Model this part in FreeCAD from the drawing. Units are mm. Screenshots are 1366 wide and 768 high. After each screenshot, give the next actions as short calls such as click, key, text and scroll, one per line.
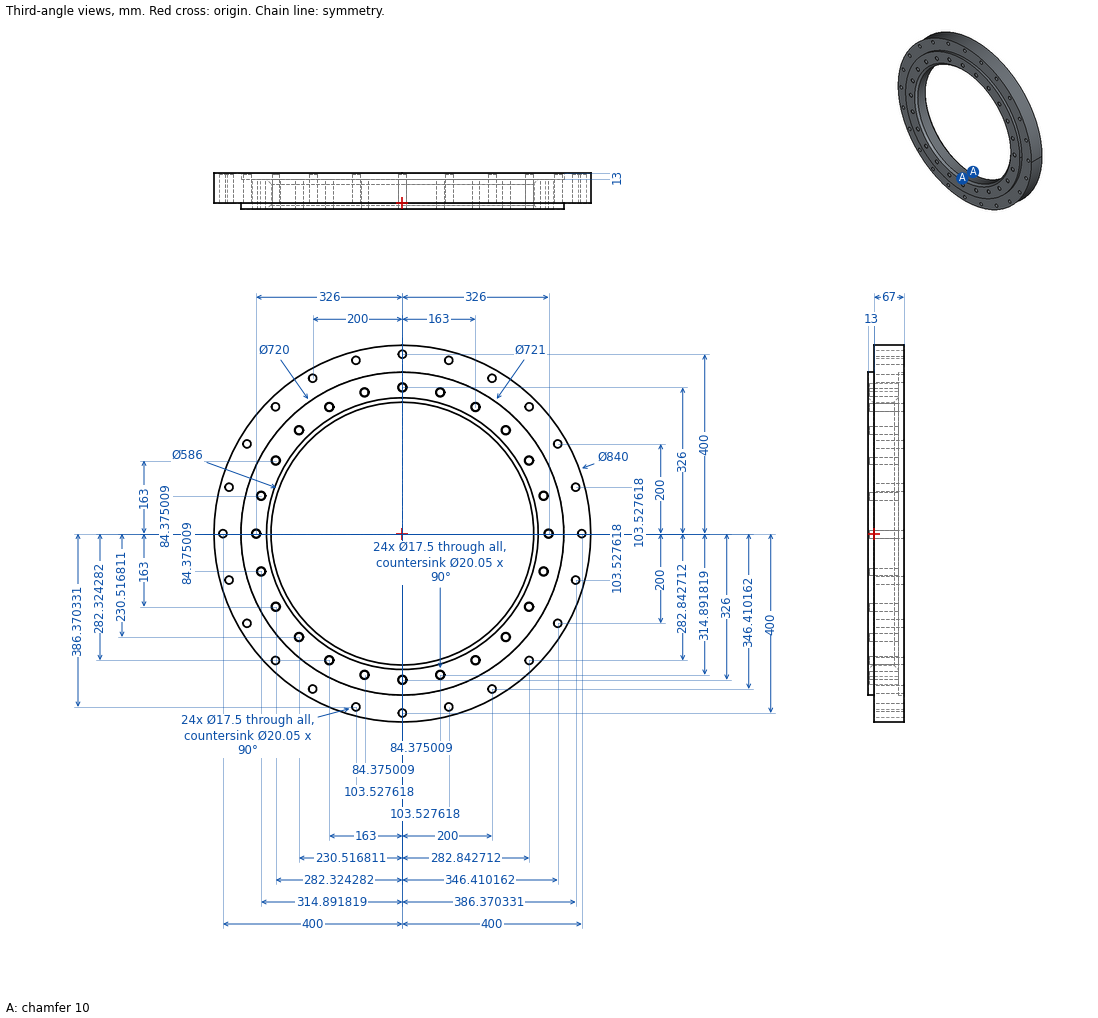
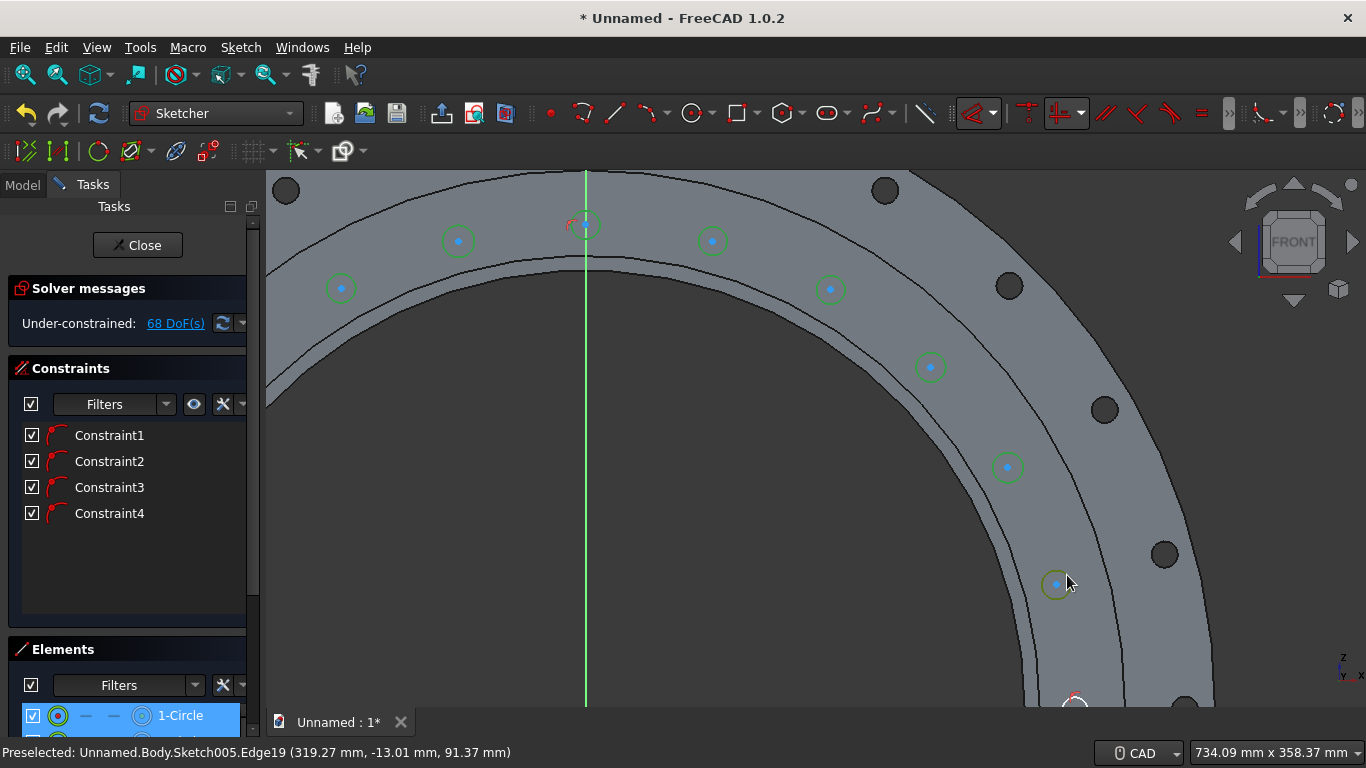
scroll(842, 281, down, 5)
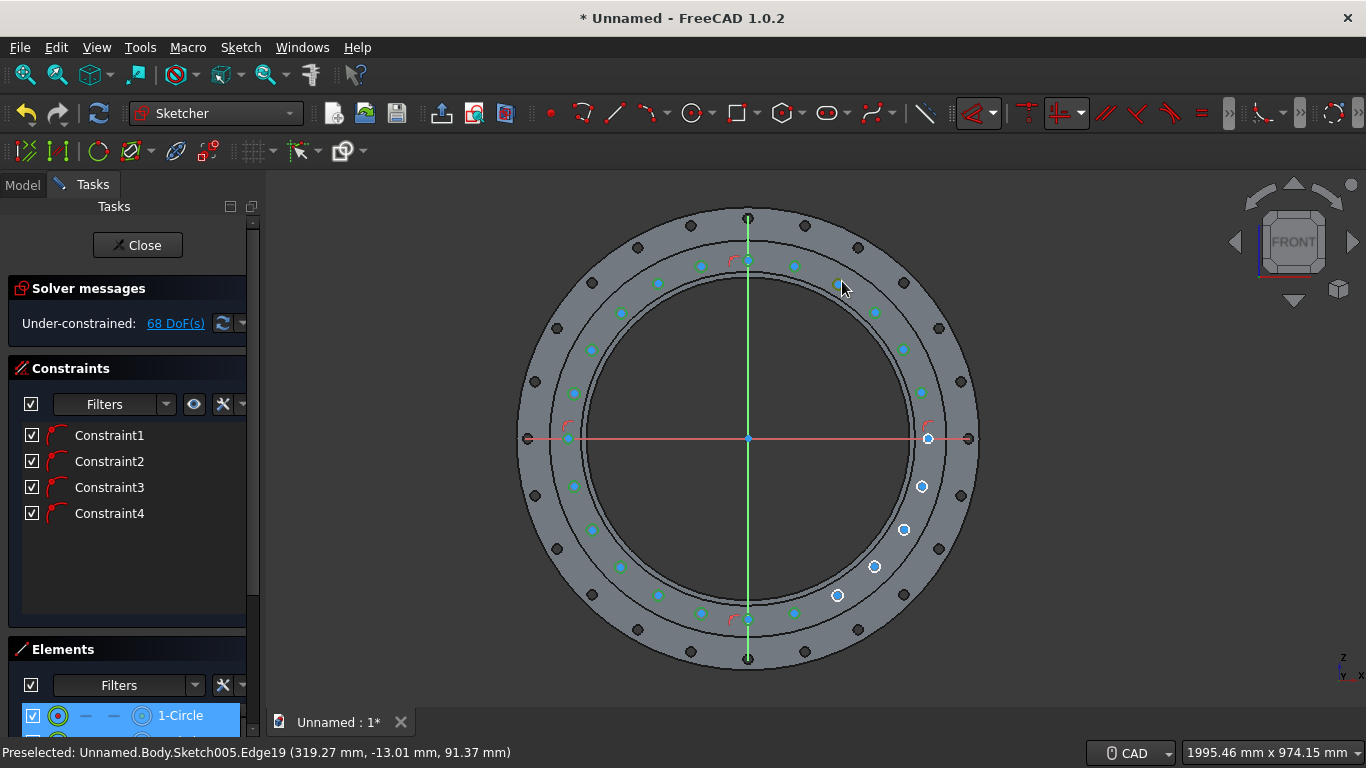
scroll(928, 434, up, 6)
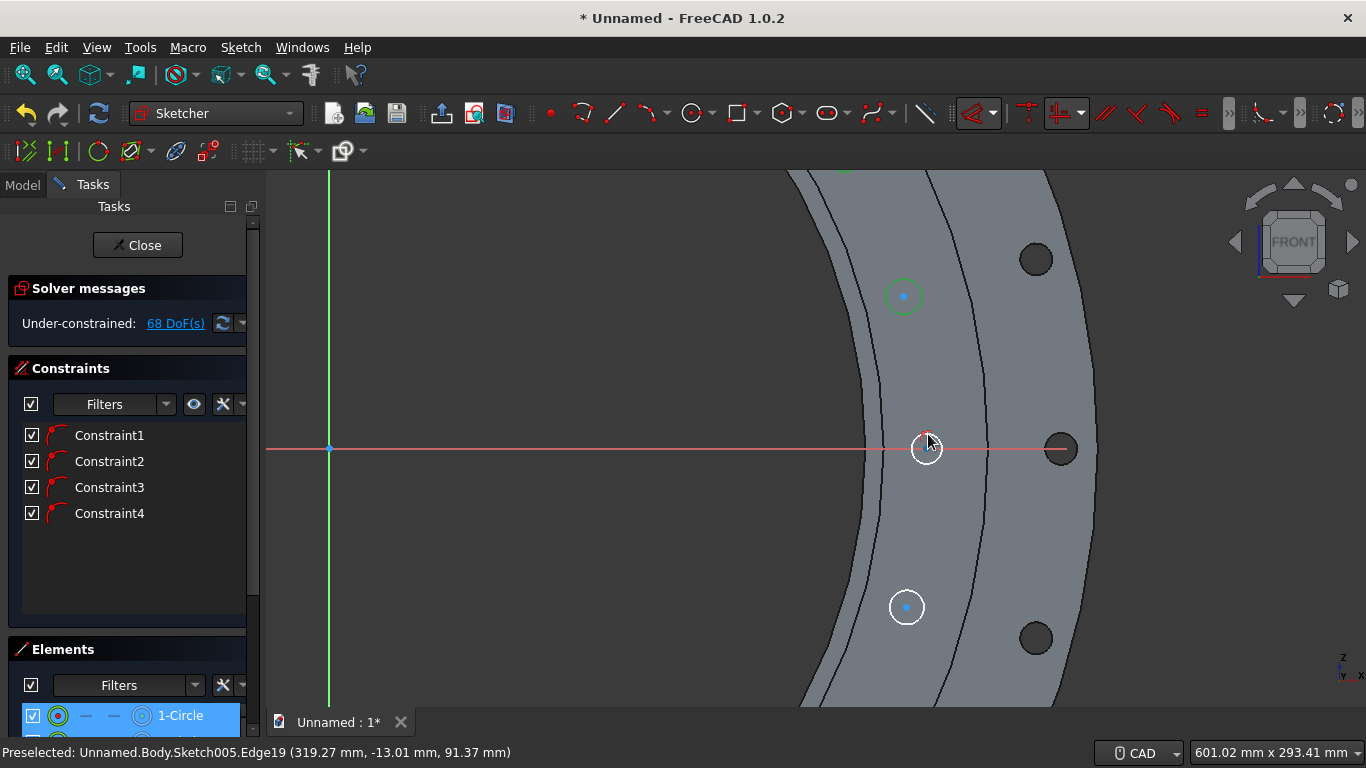
click(912, 448)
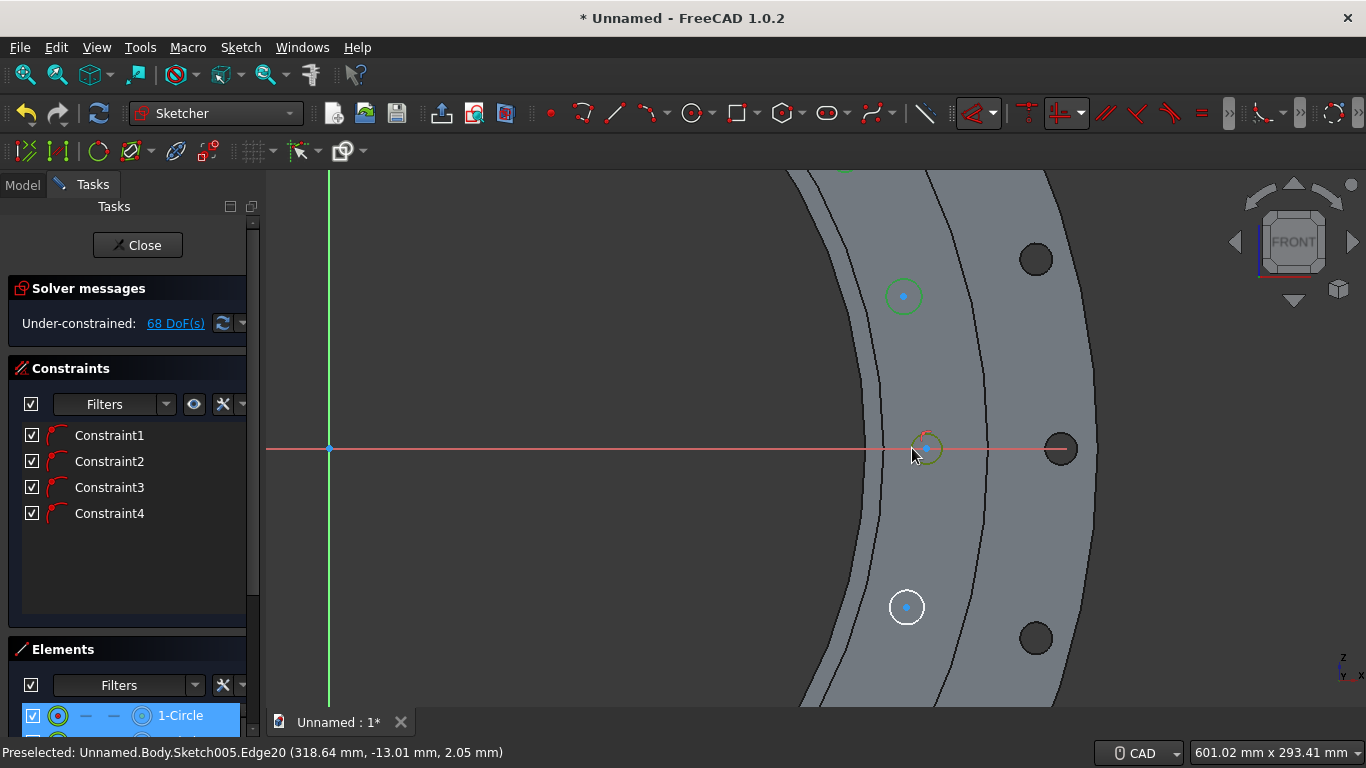
click(919, 595)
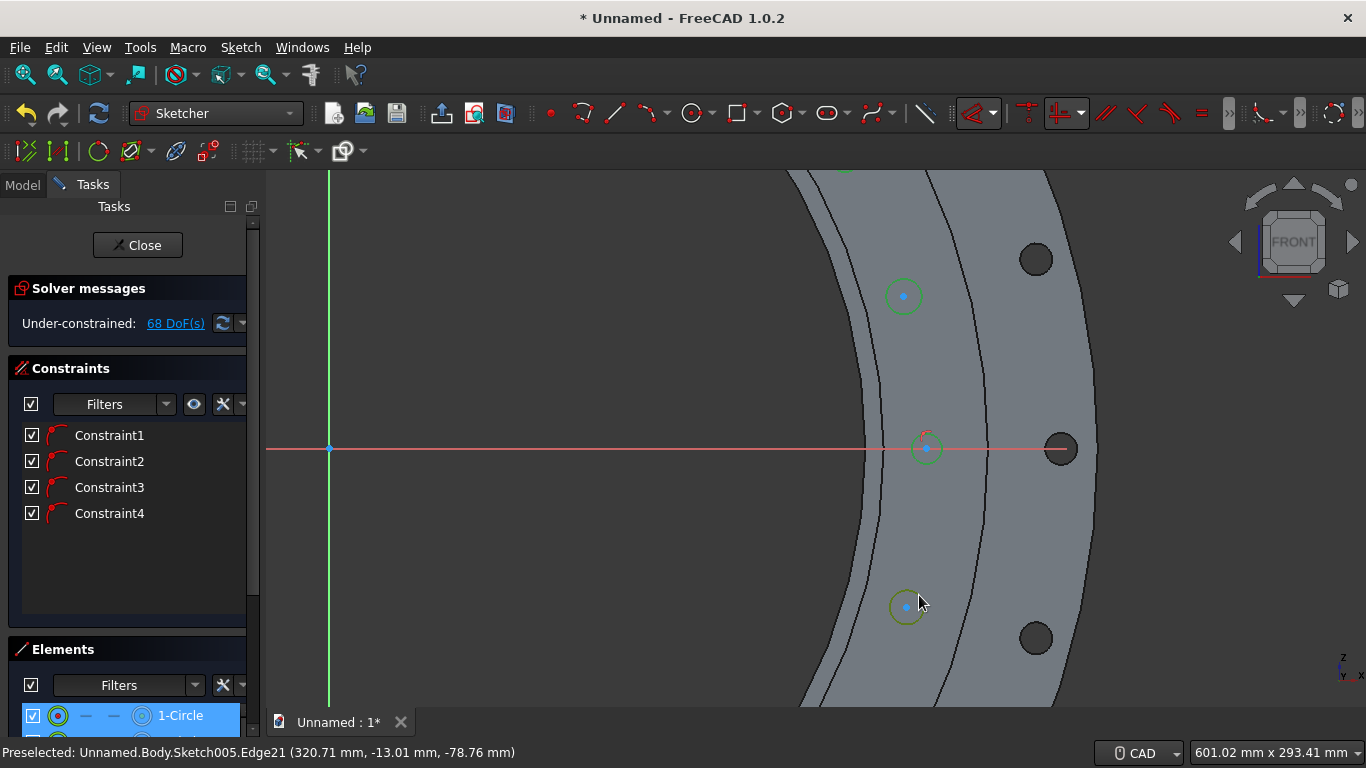
scroll(928, 434, down, 6)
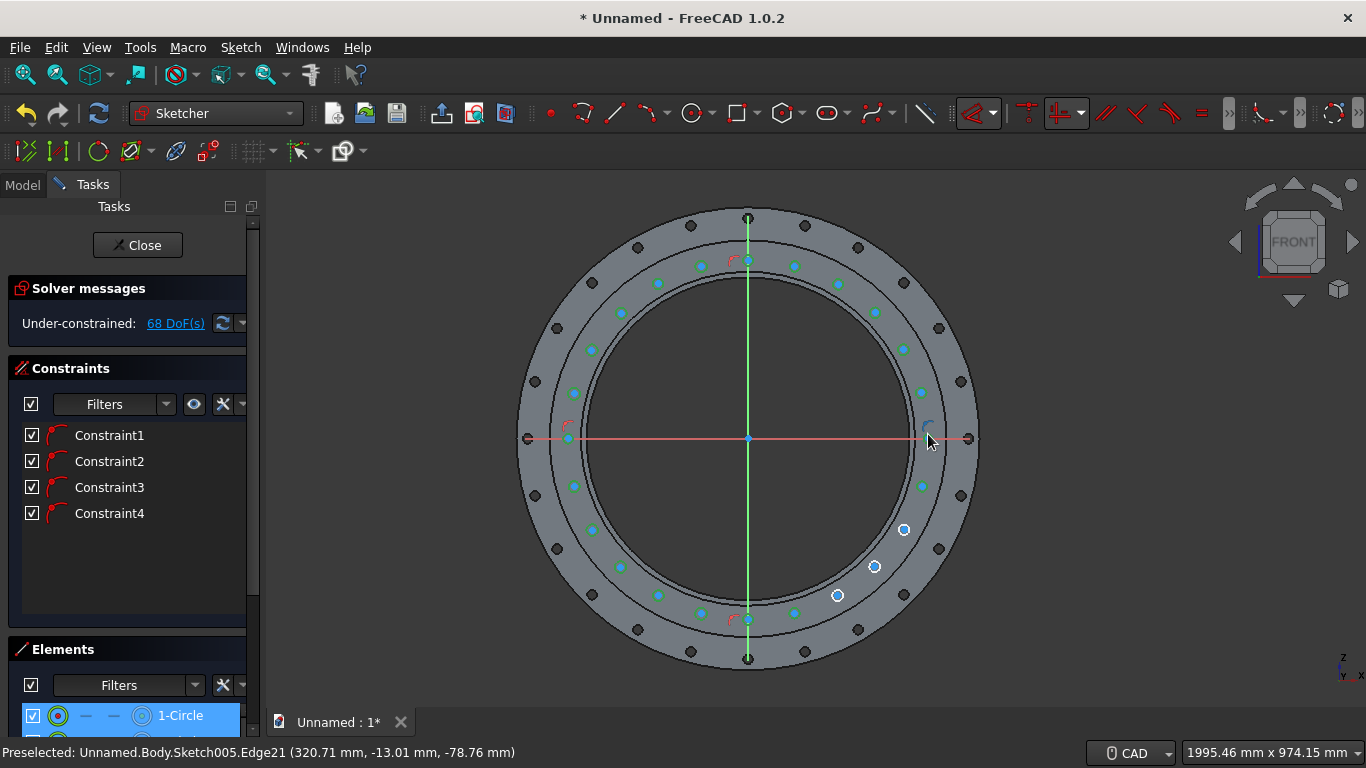
scroll(908, 526, up, 5)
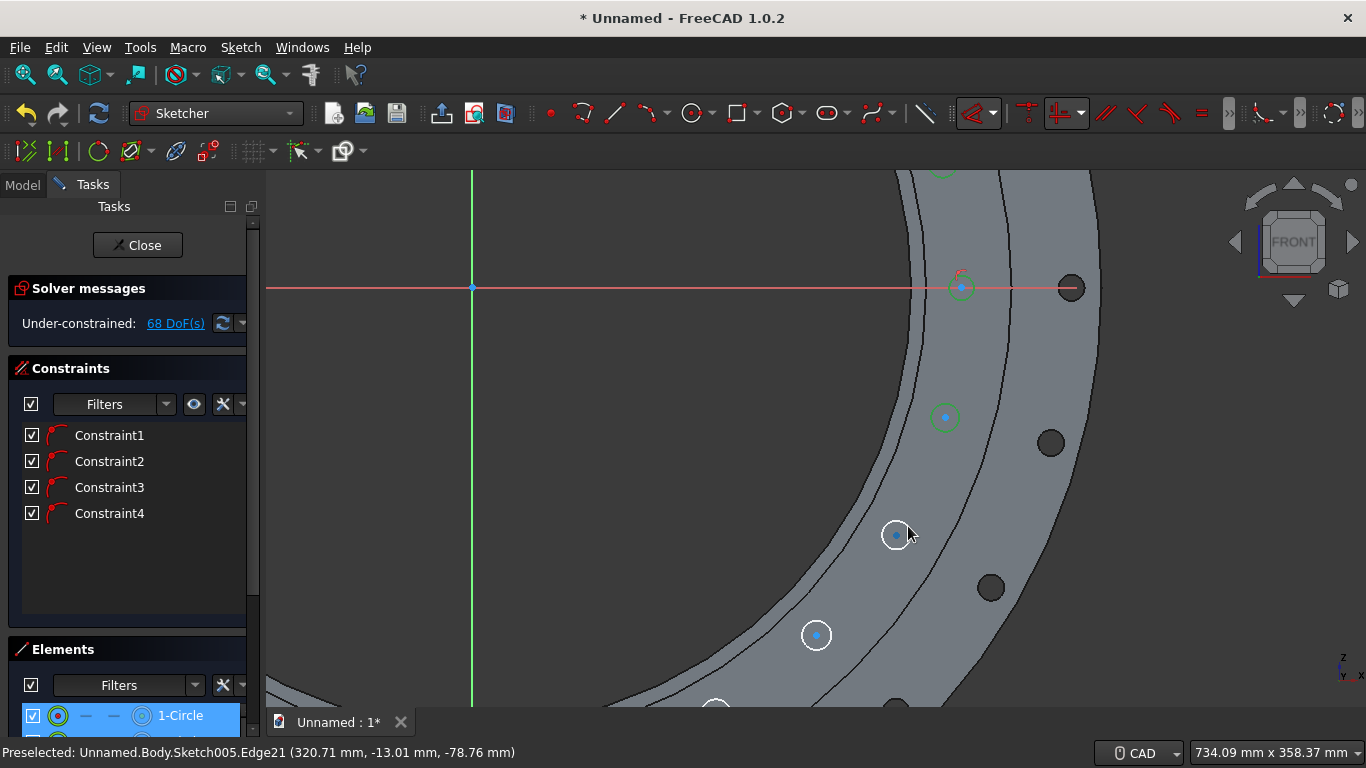
click(906, 525)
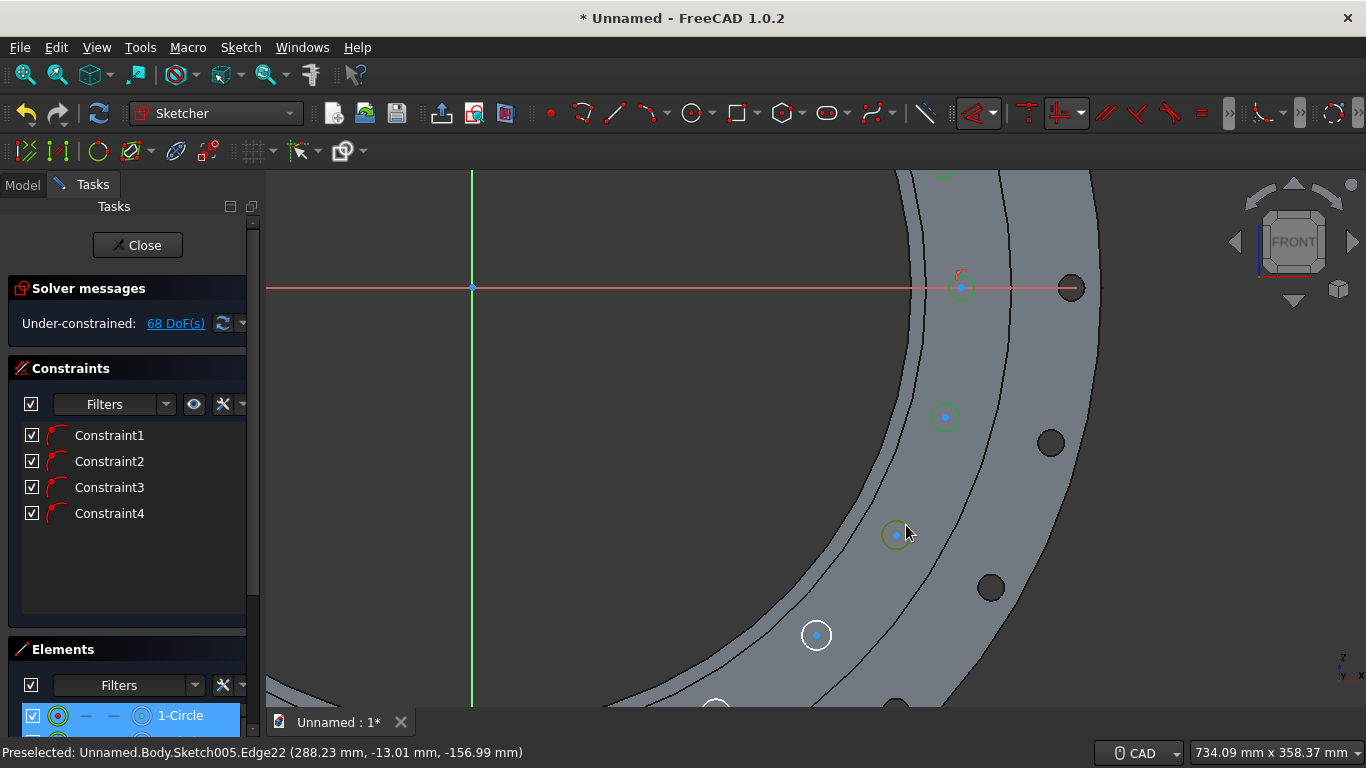
click(827, 625)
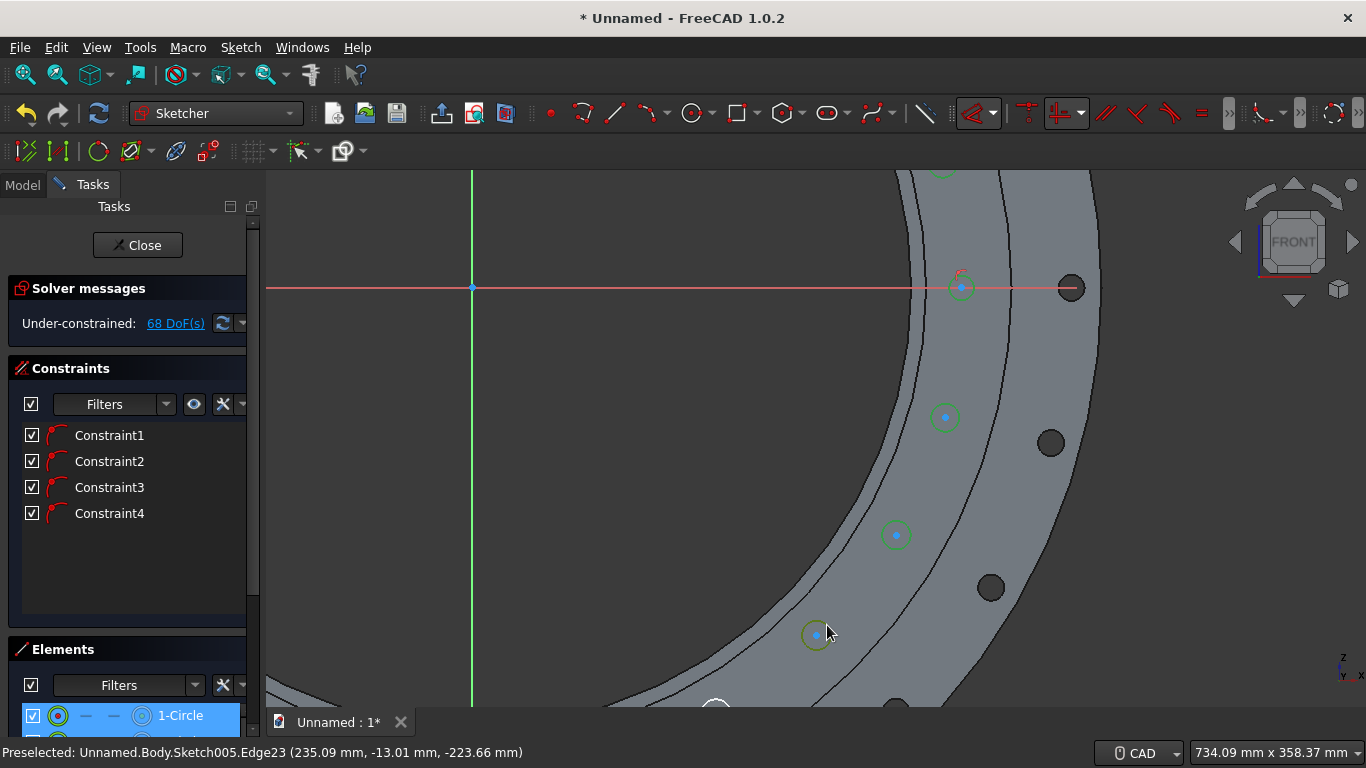
scroll(908, 526, down, 5)